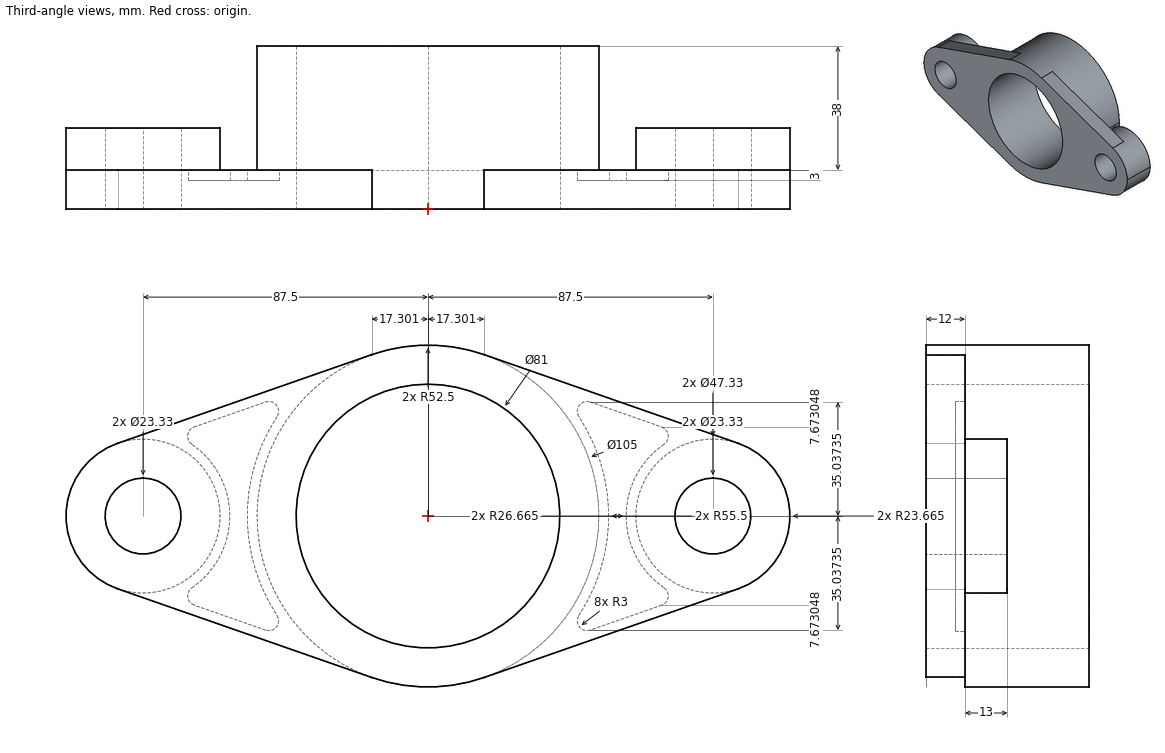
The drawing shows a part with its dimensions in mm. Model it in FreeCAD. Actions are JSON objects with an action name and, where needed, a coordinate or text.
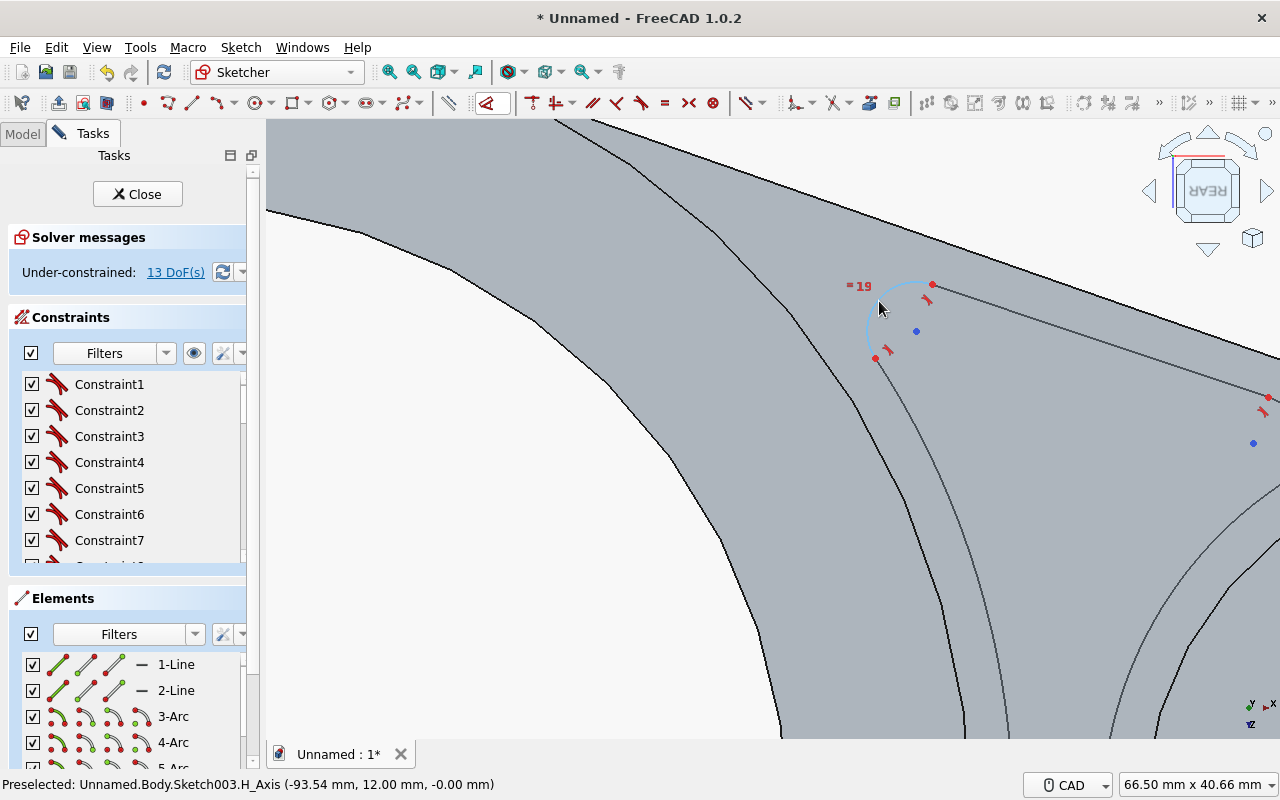
{"action": "left_click", "coordinate": [877, 301]}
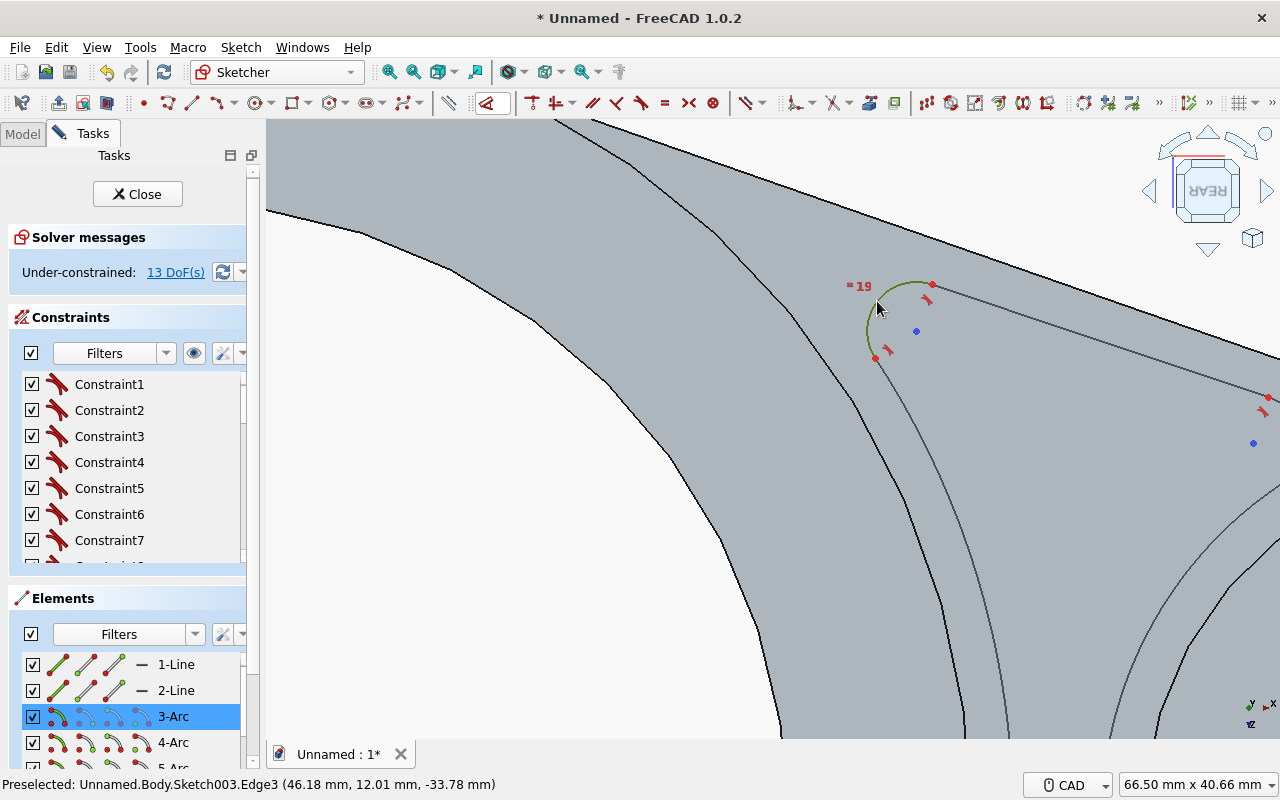
{"action": "left_click", "coordinate": [504, 104]}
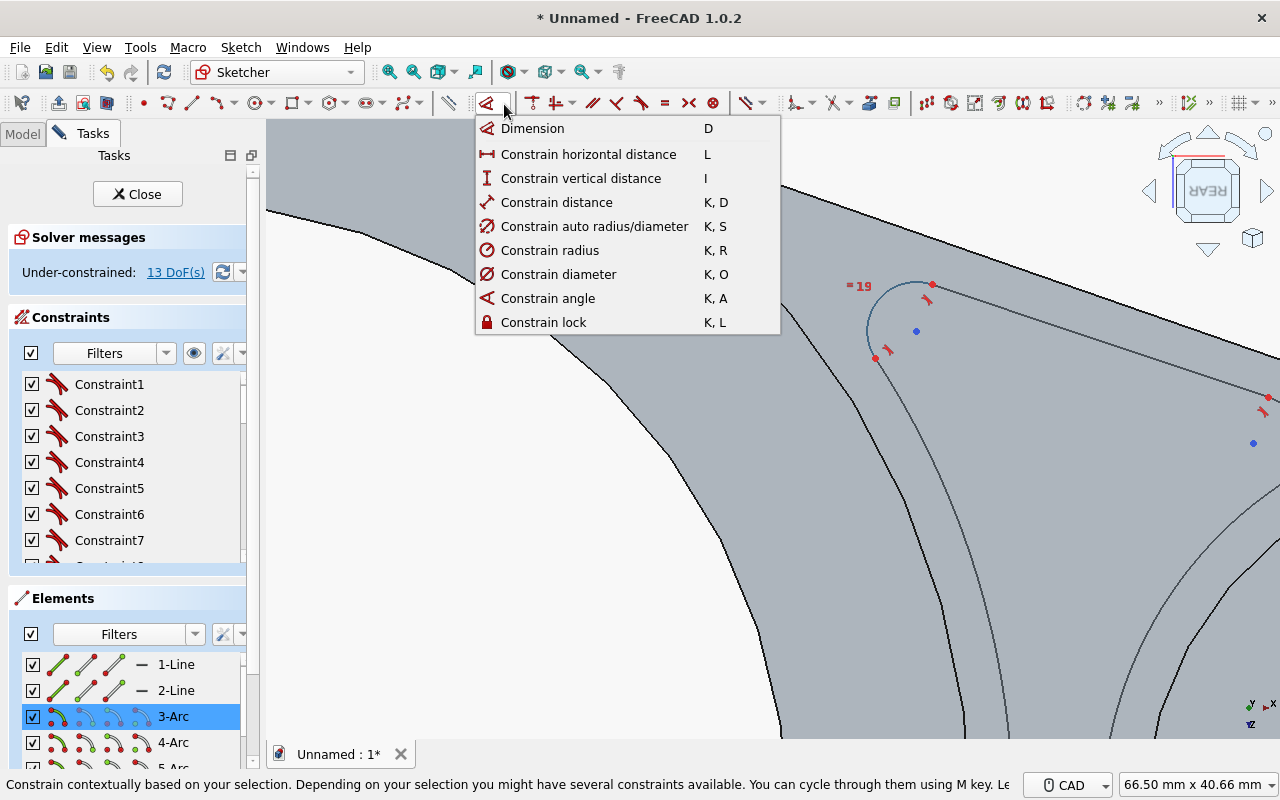
{"action": "left_click", "coordinate": [628, 250]}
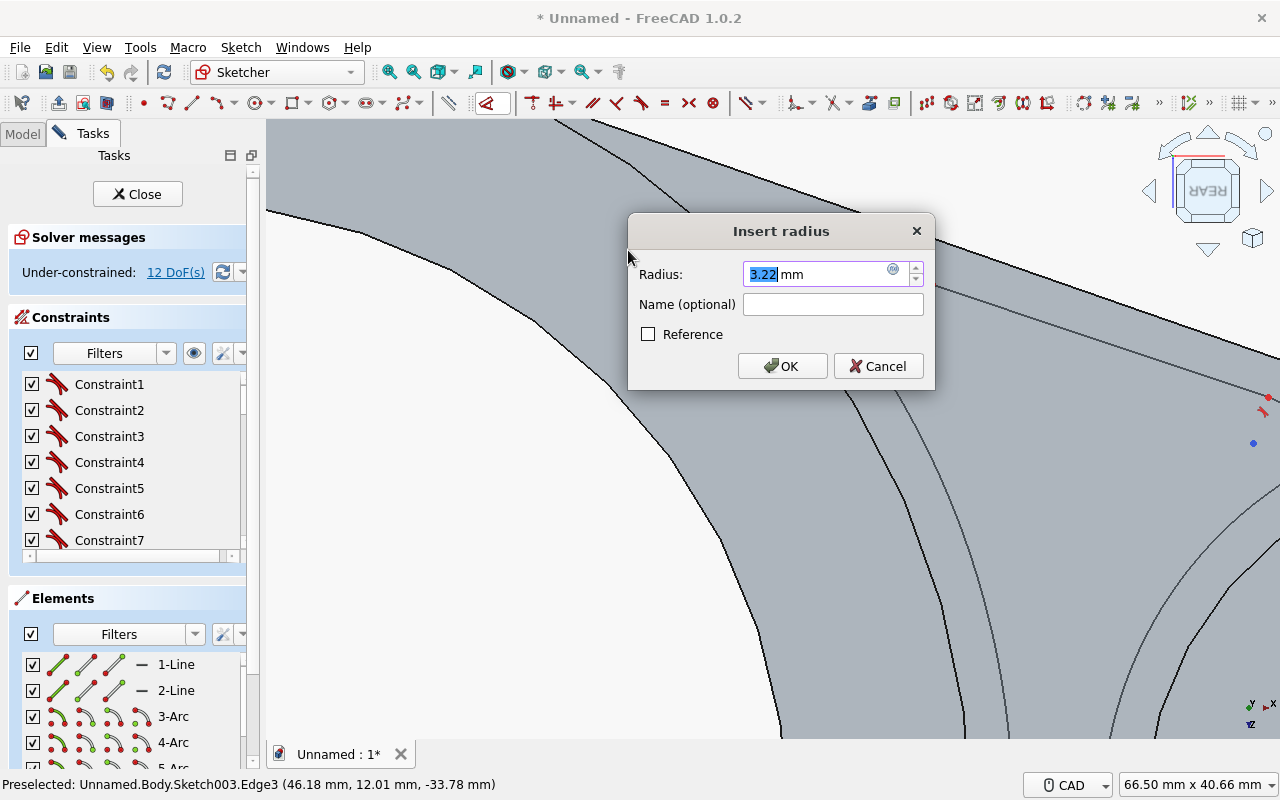
{"action": "type", "text": "3"}
{"action": "key", "text": "Return"}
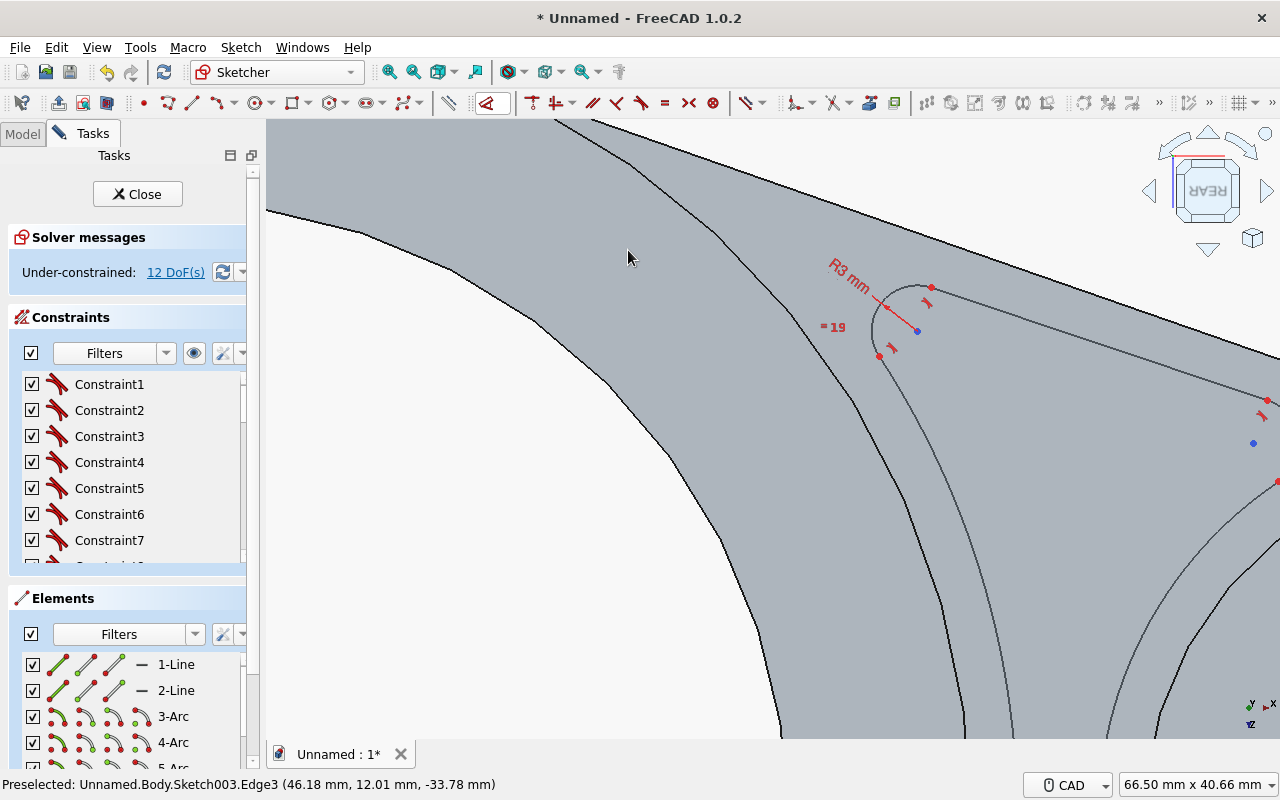
{"action": "scroll", "coordinate": [879, 301], "scroll_direction": "down", "scroll_amount": 7}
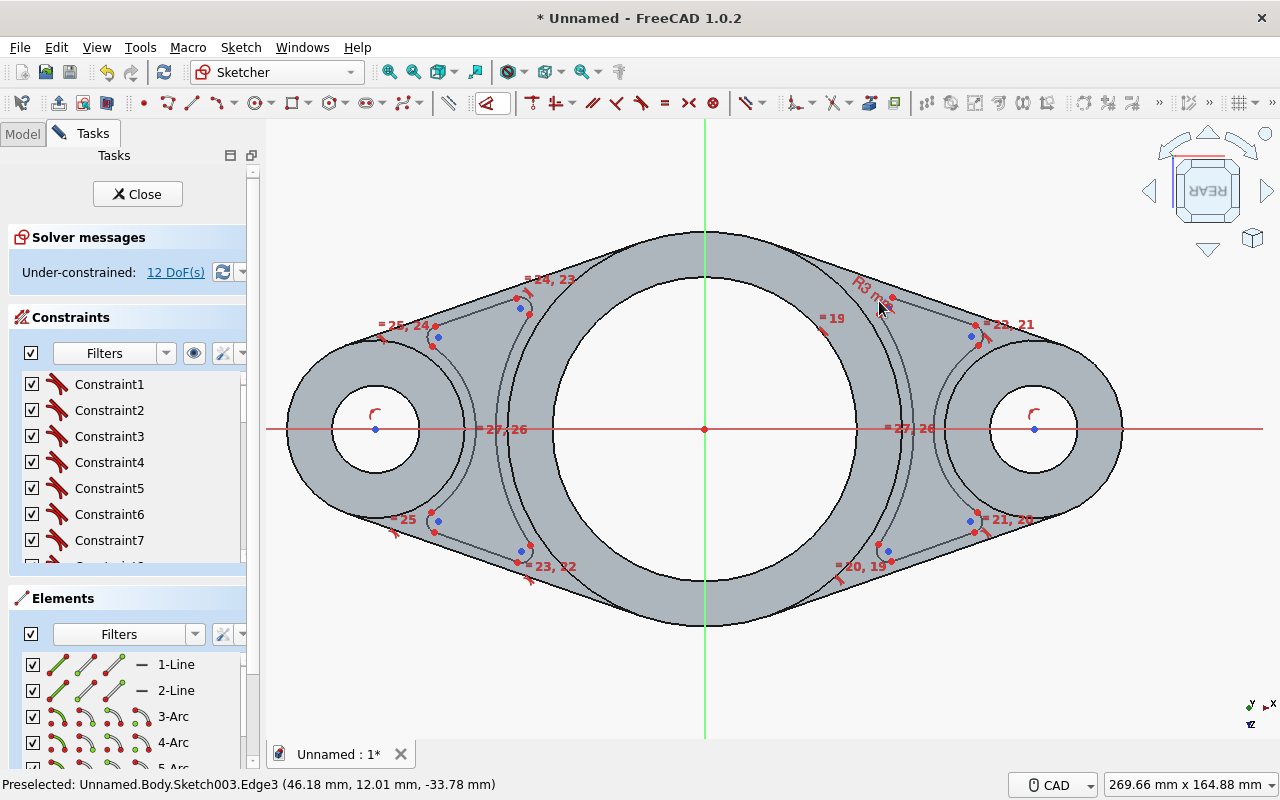
{"action": "left_click", "coordinate": [908, 382]}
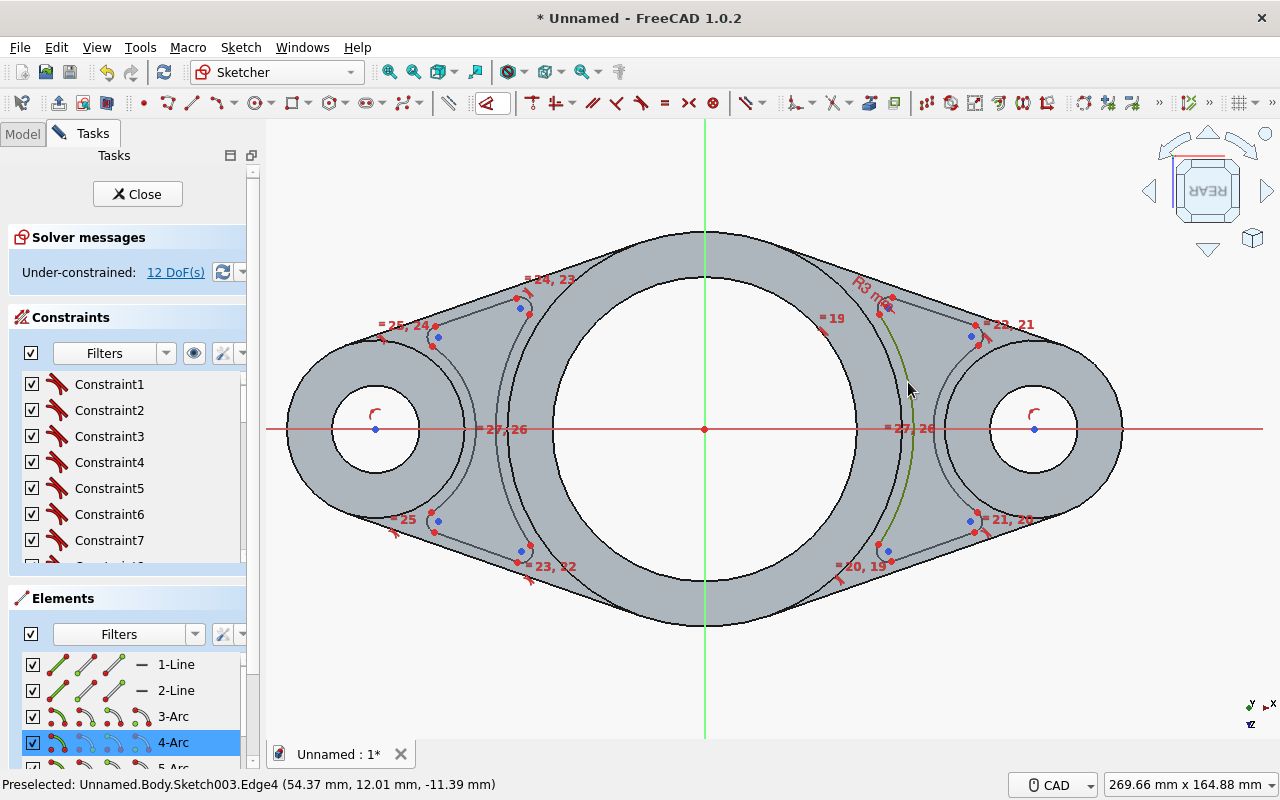
{"action": "key", "text": "k r"}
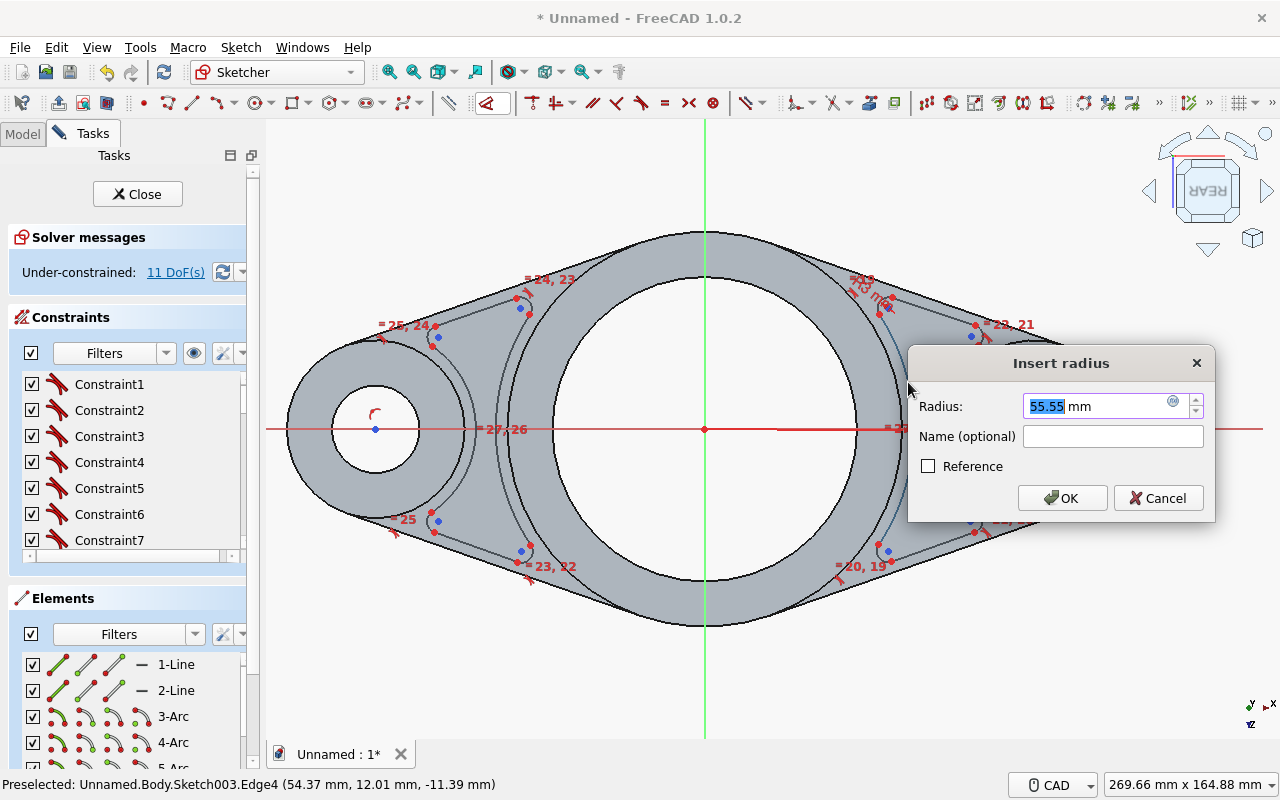
{"action": "type", "text": "55.5"}
{"action": "key", "text": "Return"}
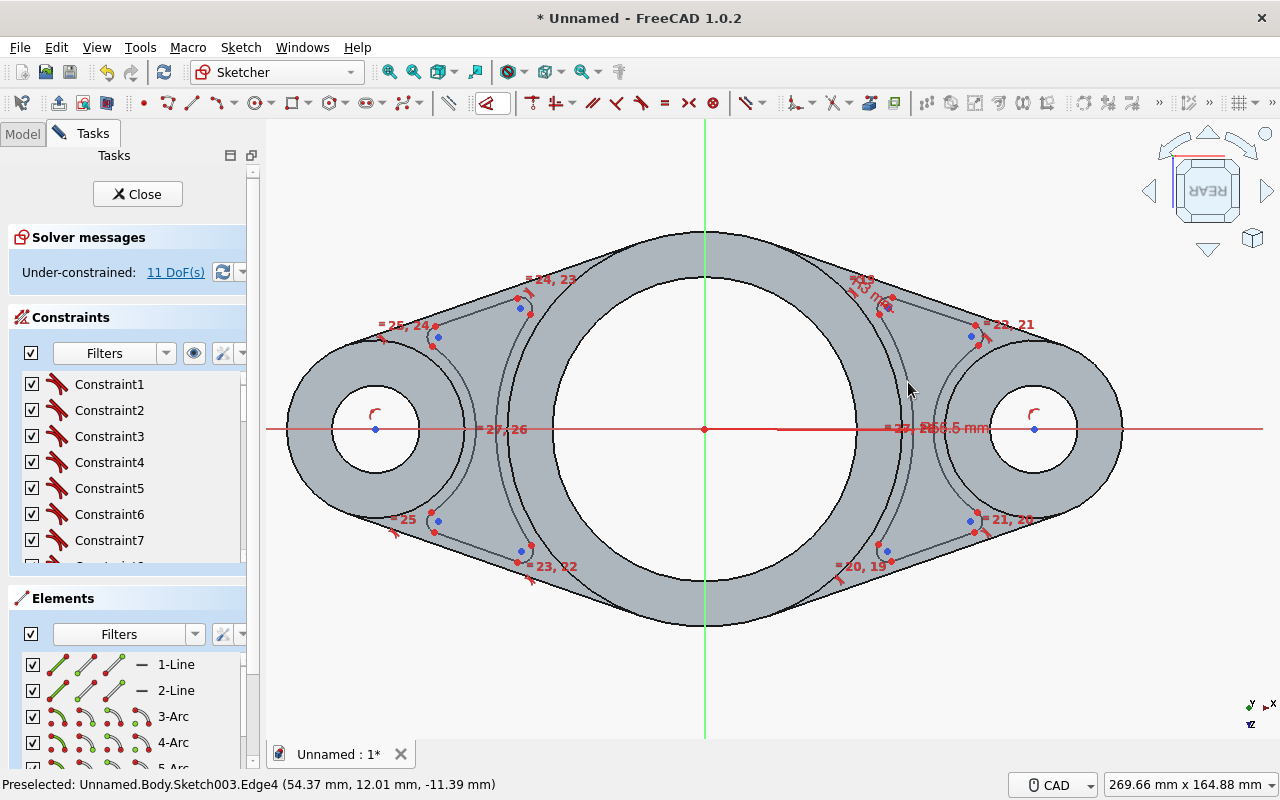
{"action": "left_click", "coordinate": [941, 391]}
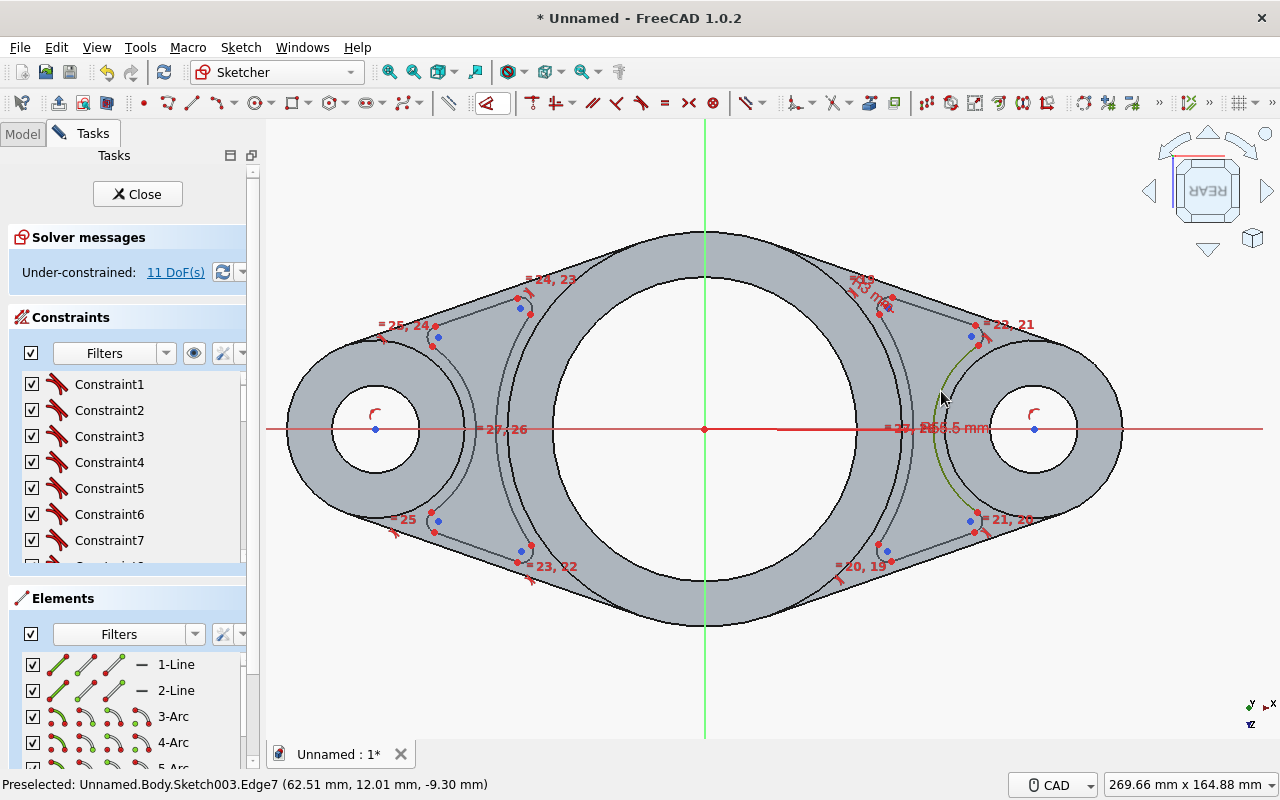
{"action": "key", "text": "k r"}